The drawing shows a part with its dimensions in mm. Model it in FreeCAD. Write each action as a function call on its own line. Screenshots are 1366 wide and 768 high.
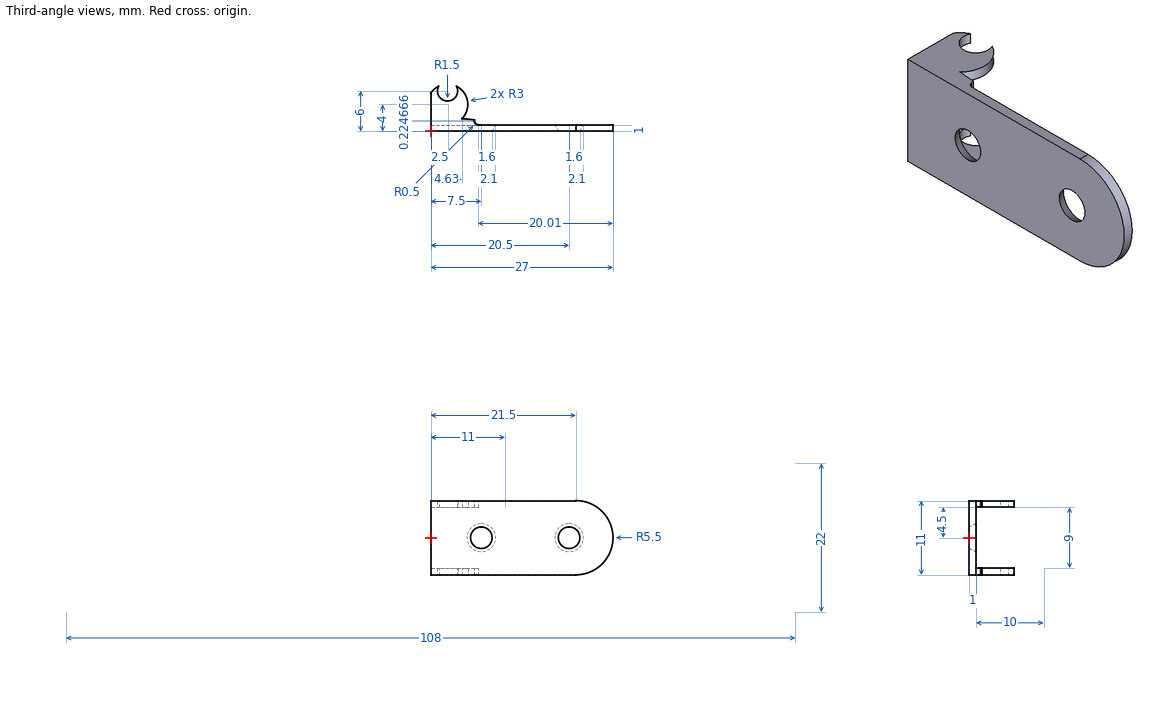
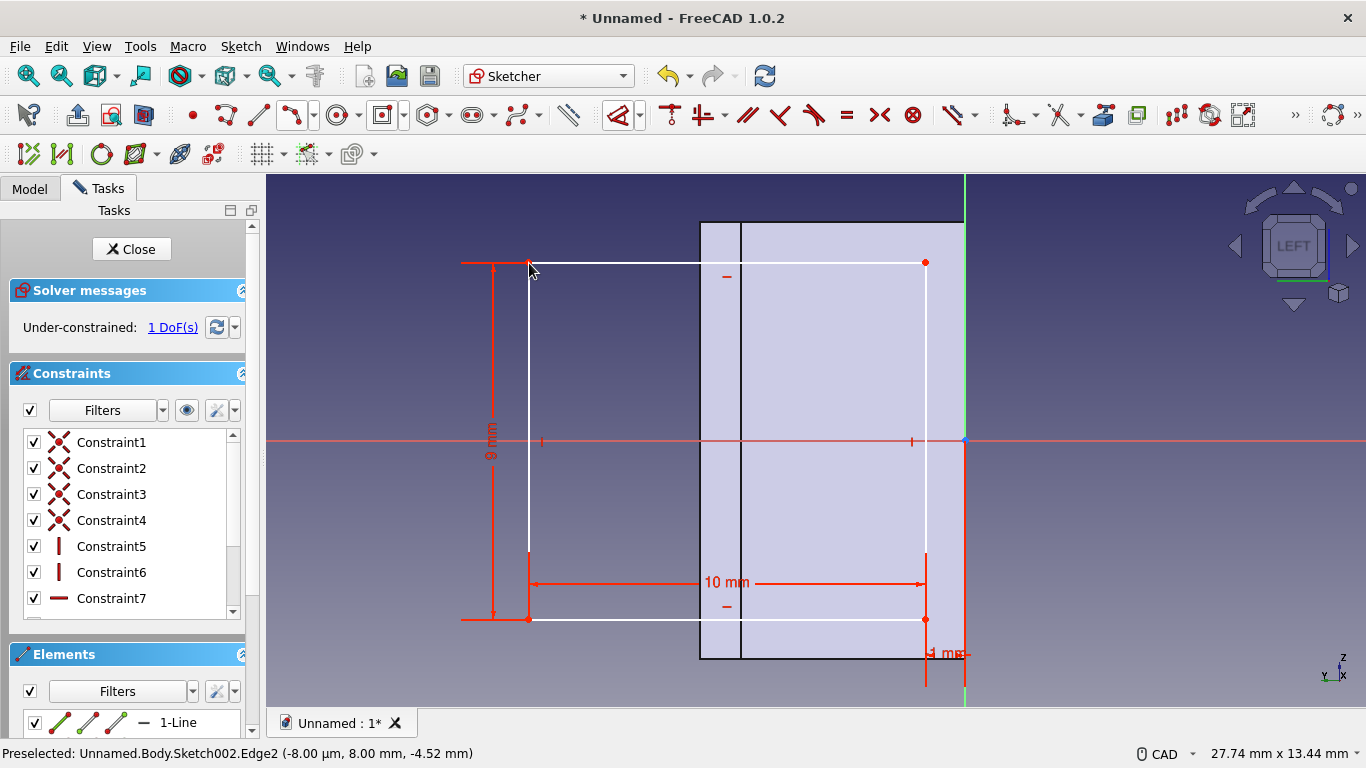
key(i)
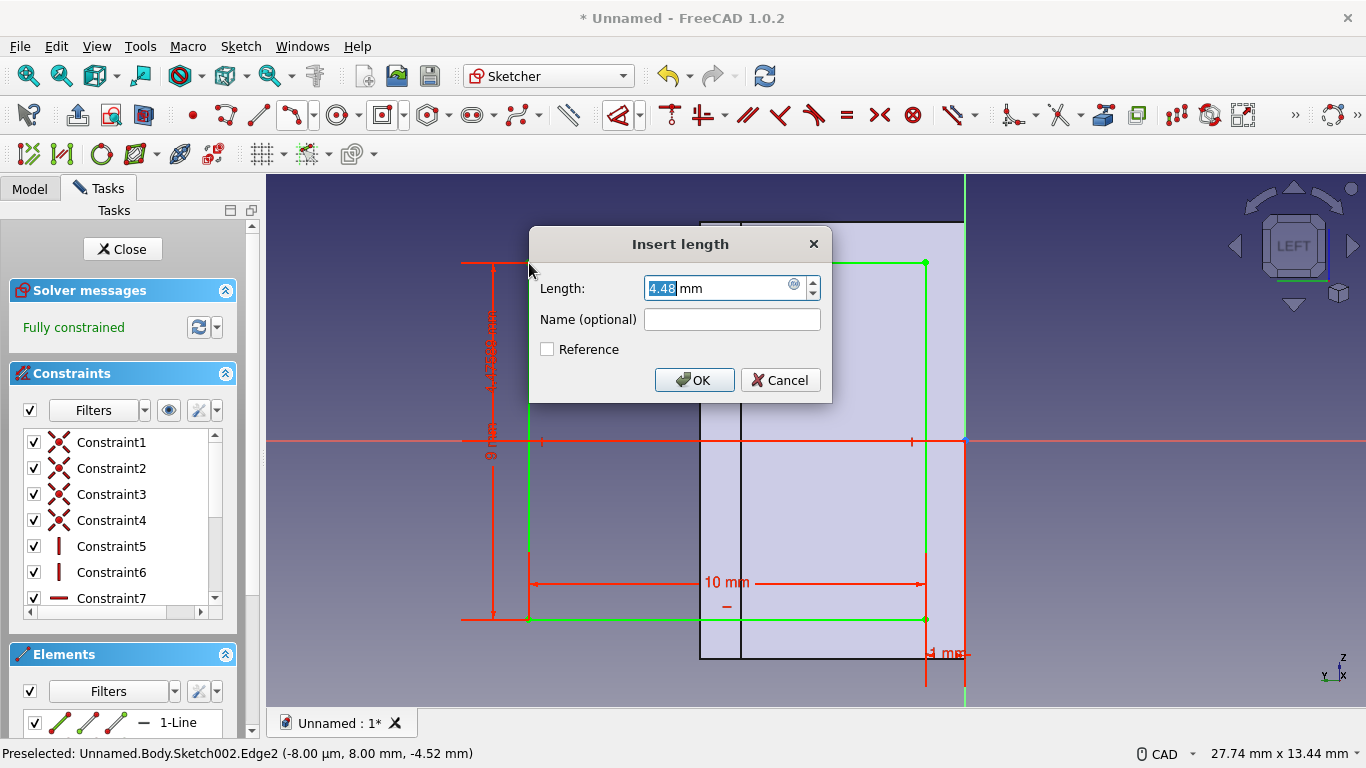
text(4.5)
key(Return)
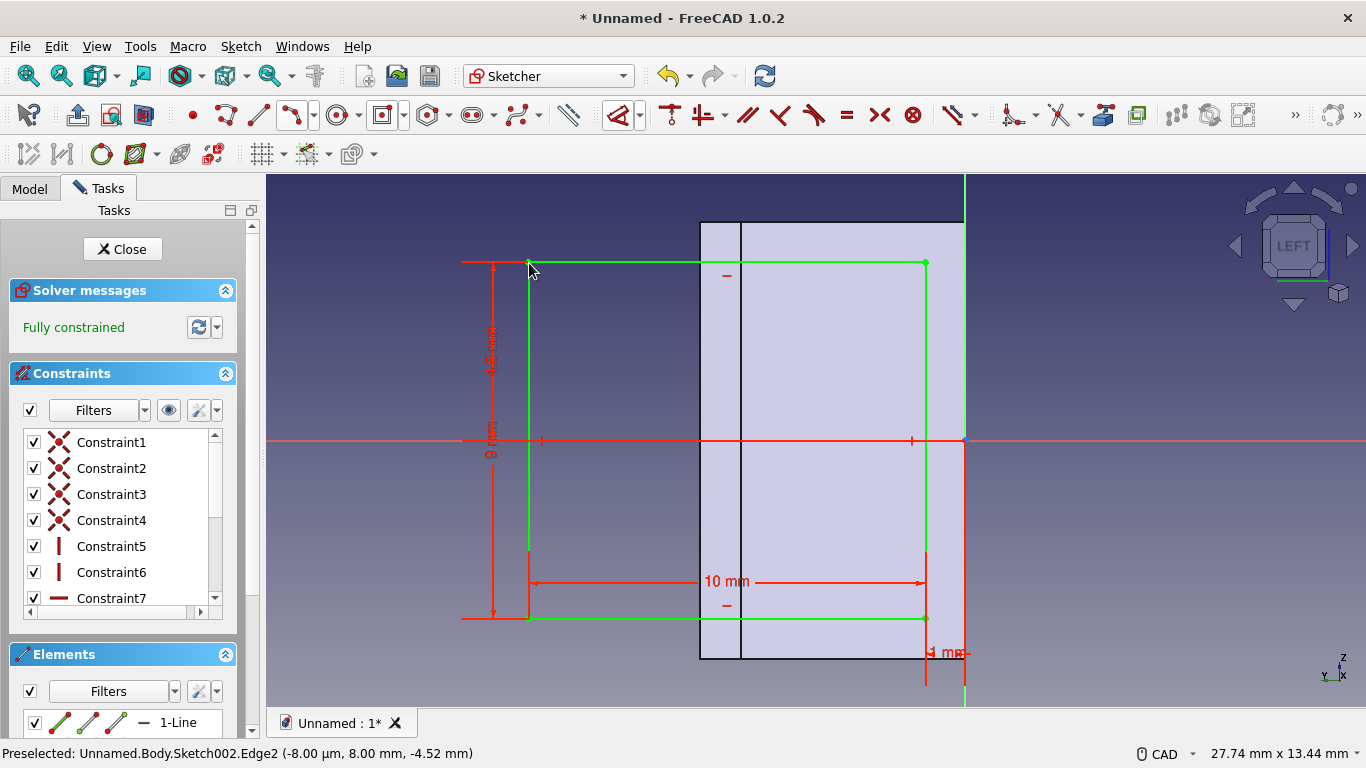
click(123, 249)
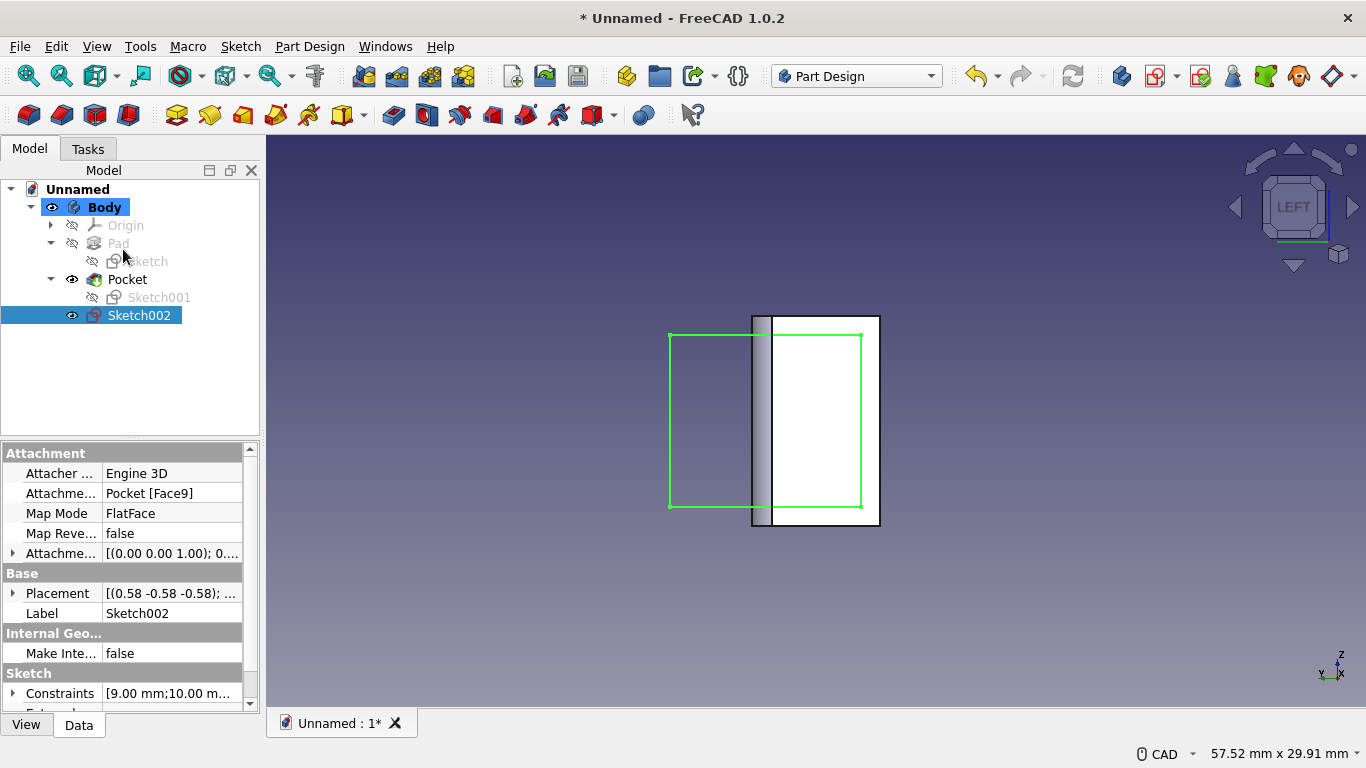
click(394, 116)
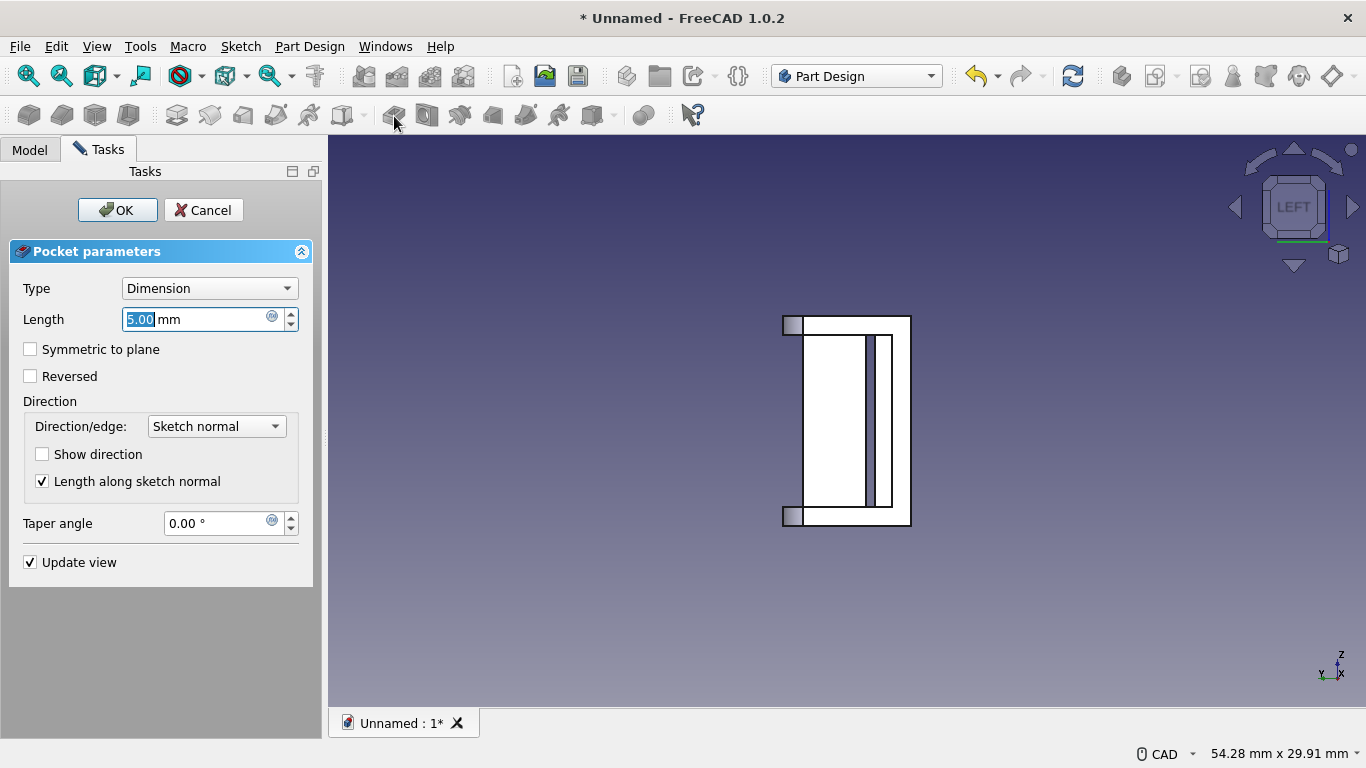
text(11)
key(Tab)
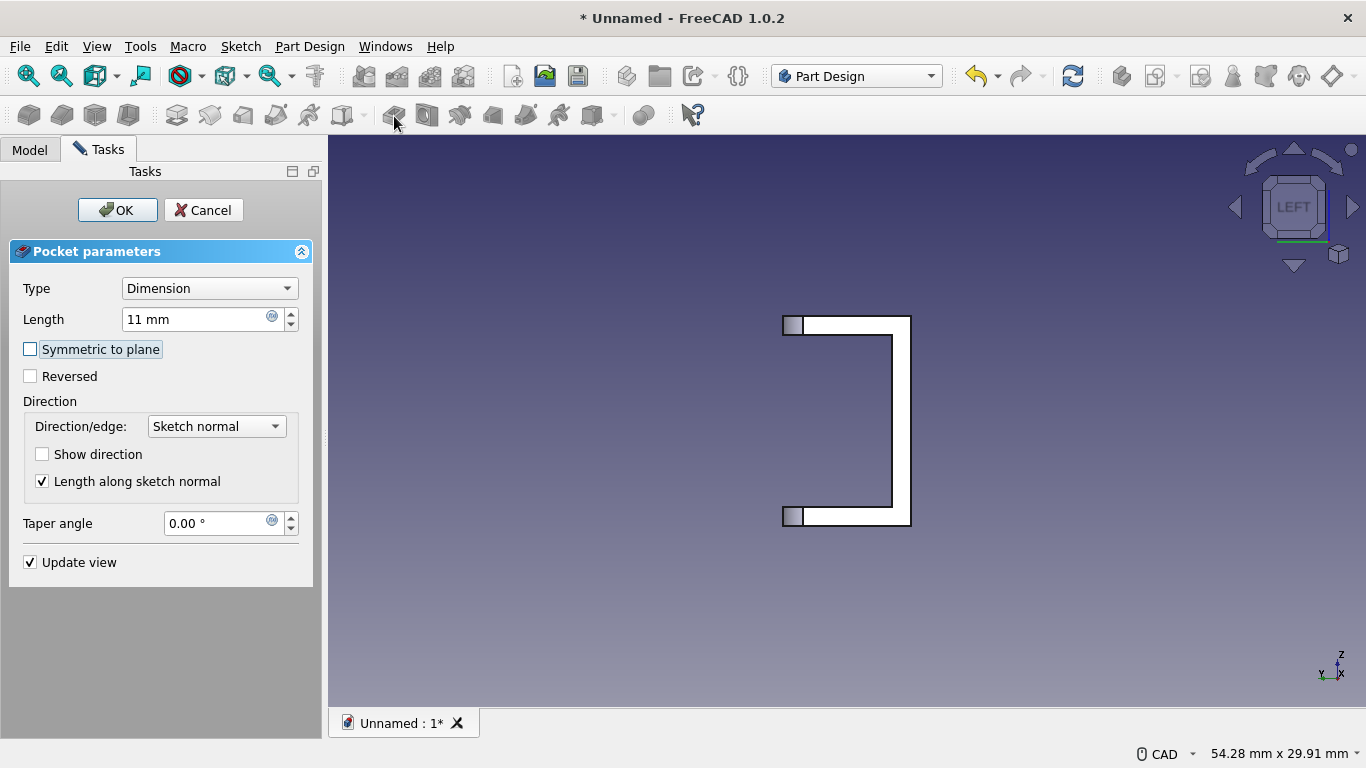
click(118, 210)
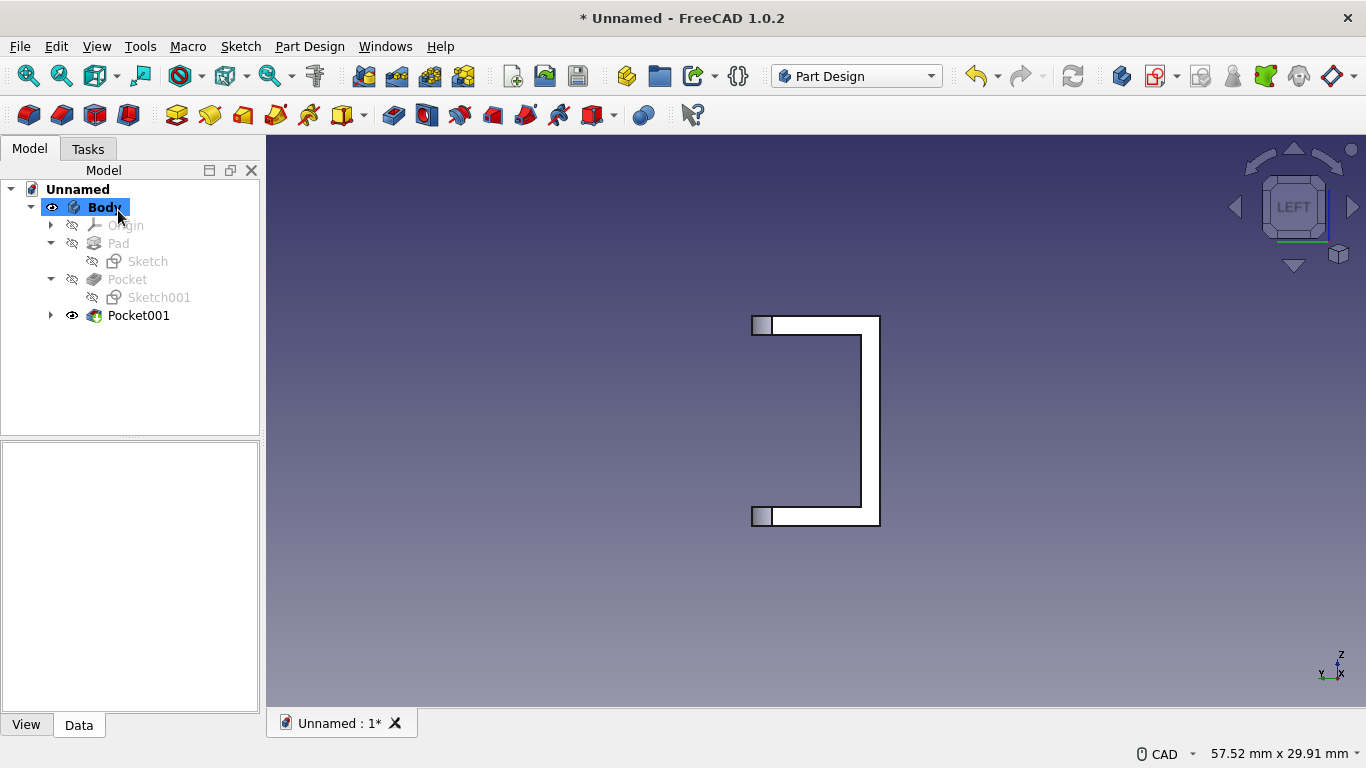
click(29, 76)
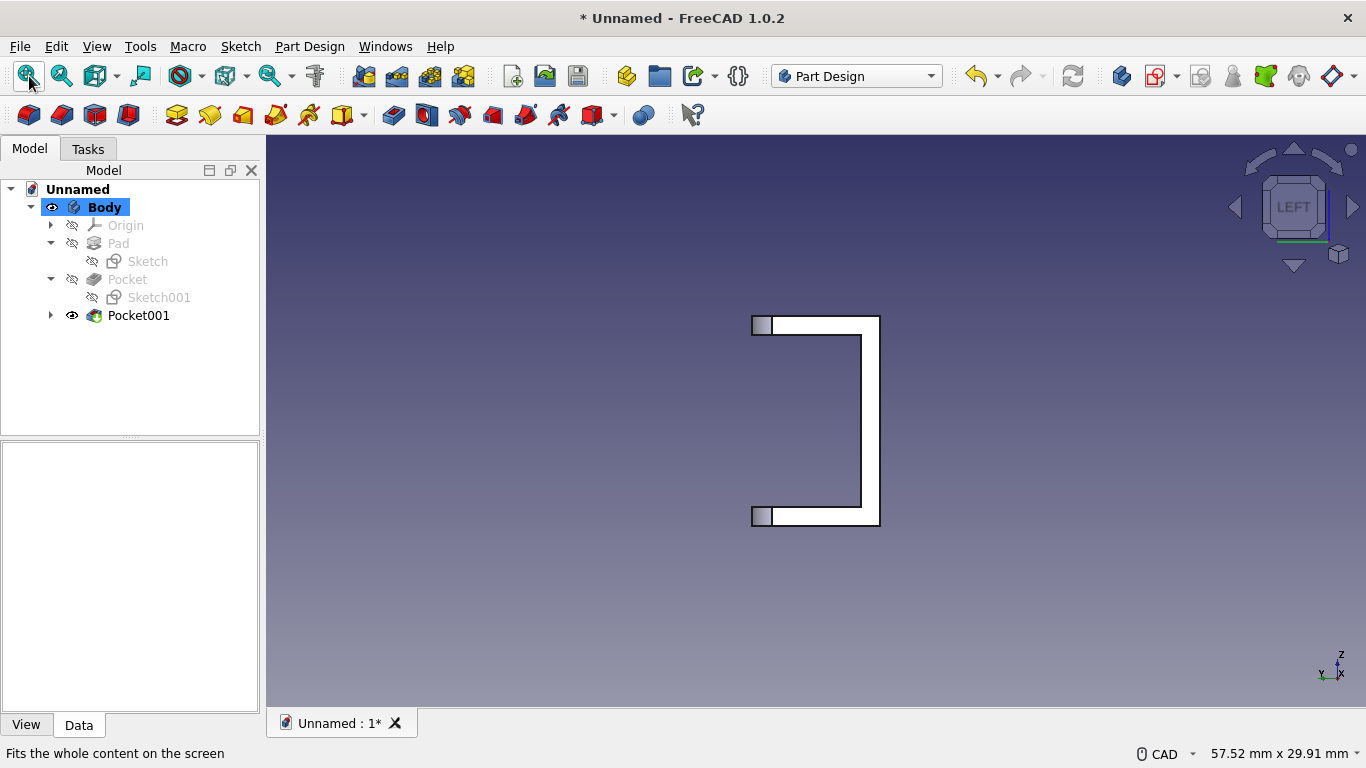
click(1154, 76)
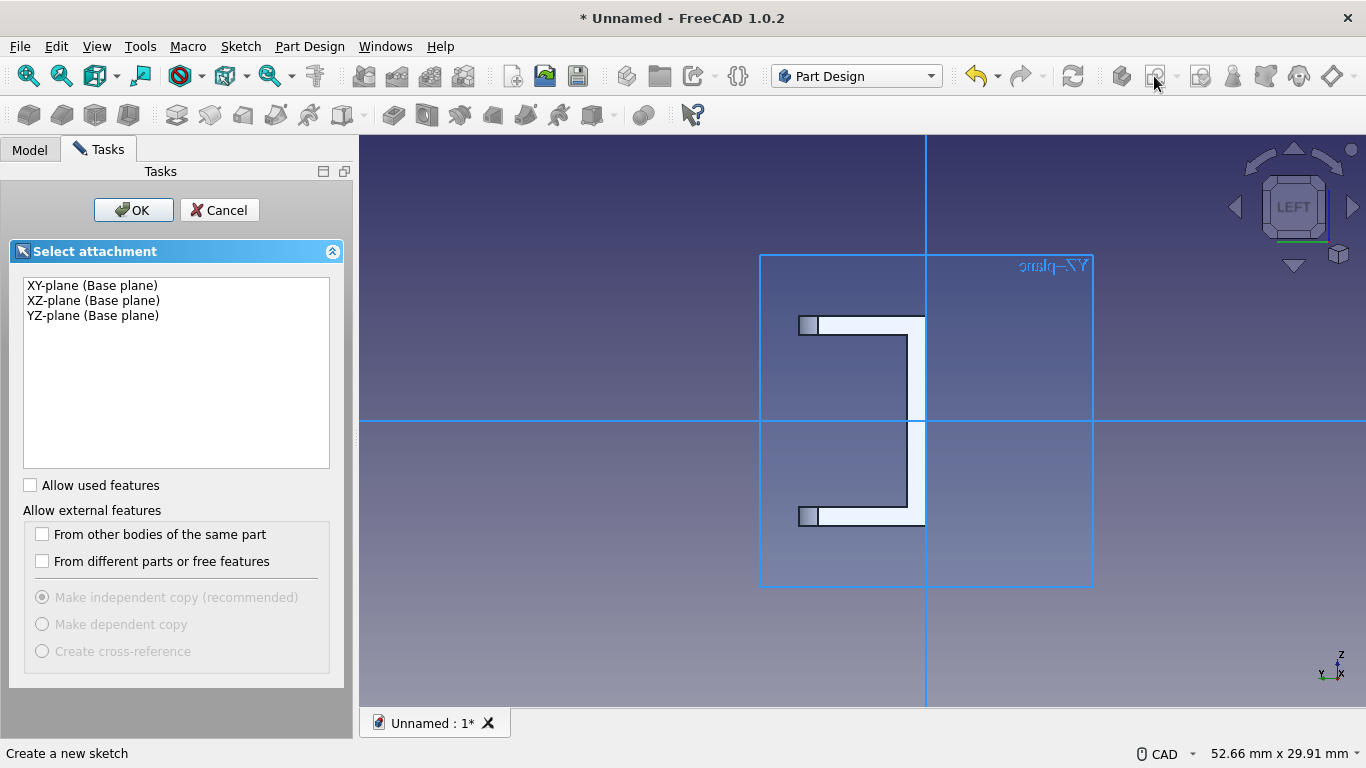
click(84, 286)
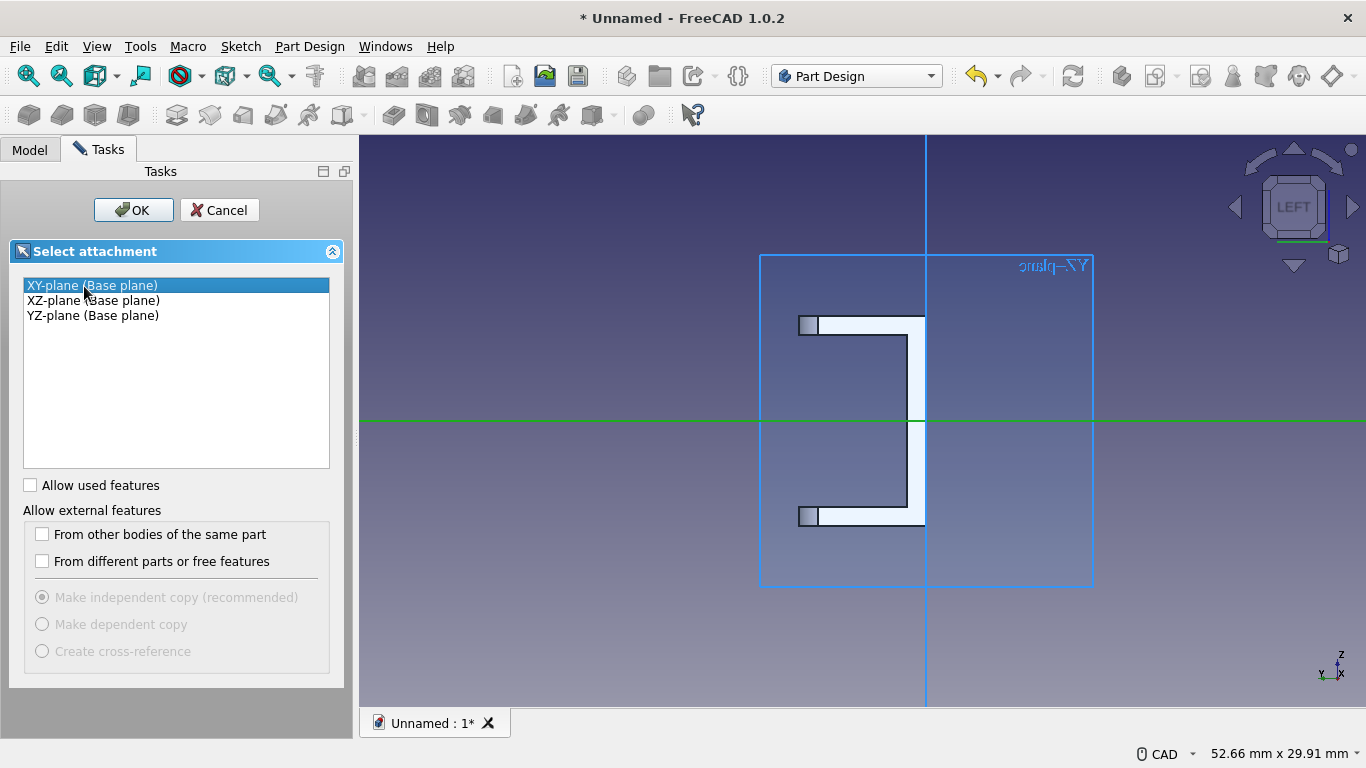
click(134, 210)